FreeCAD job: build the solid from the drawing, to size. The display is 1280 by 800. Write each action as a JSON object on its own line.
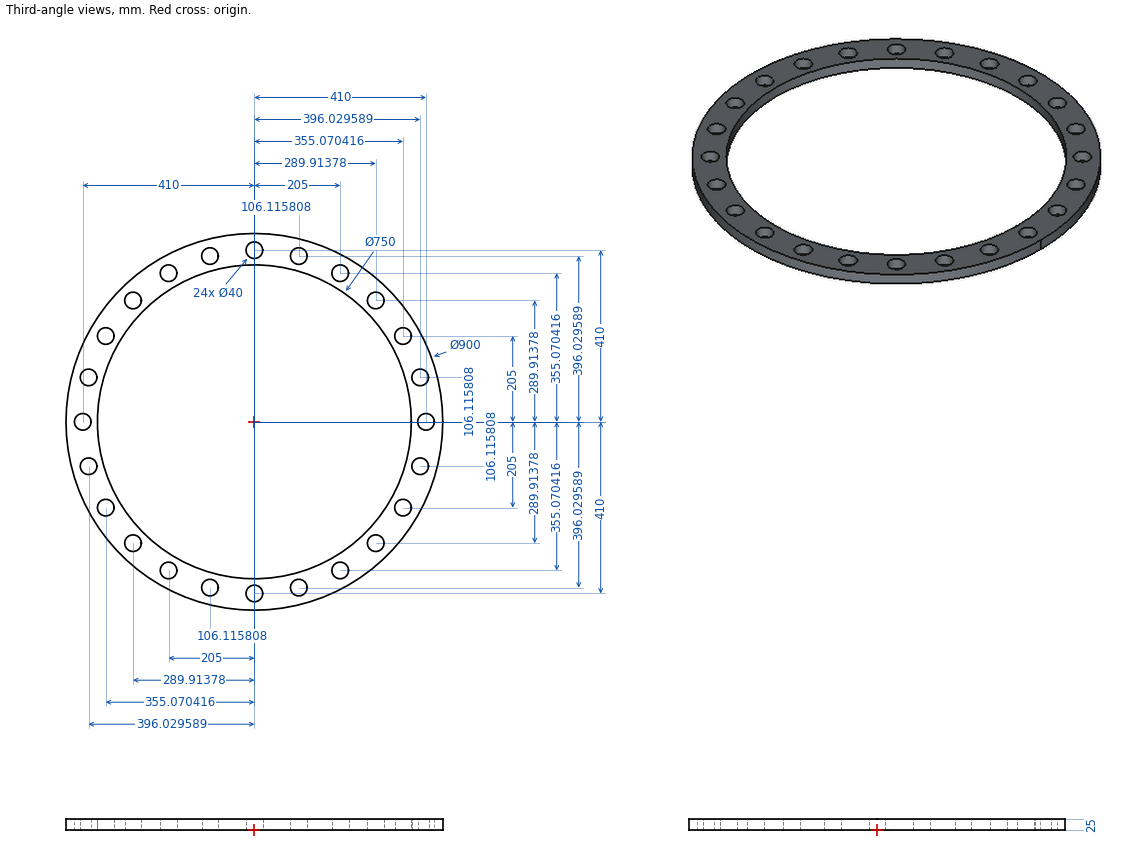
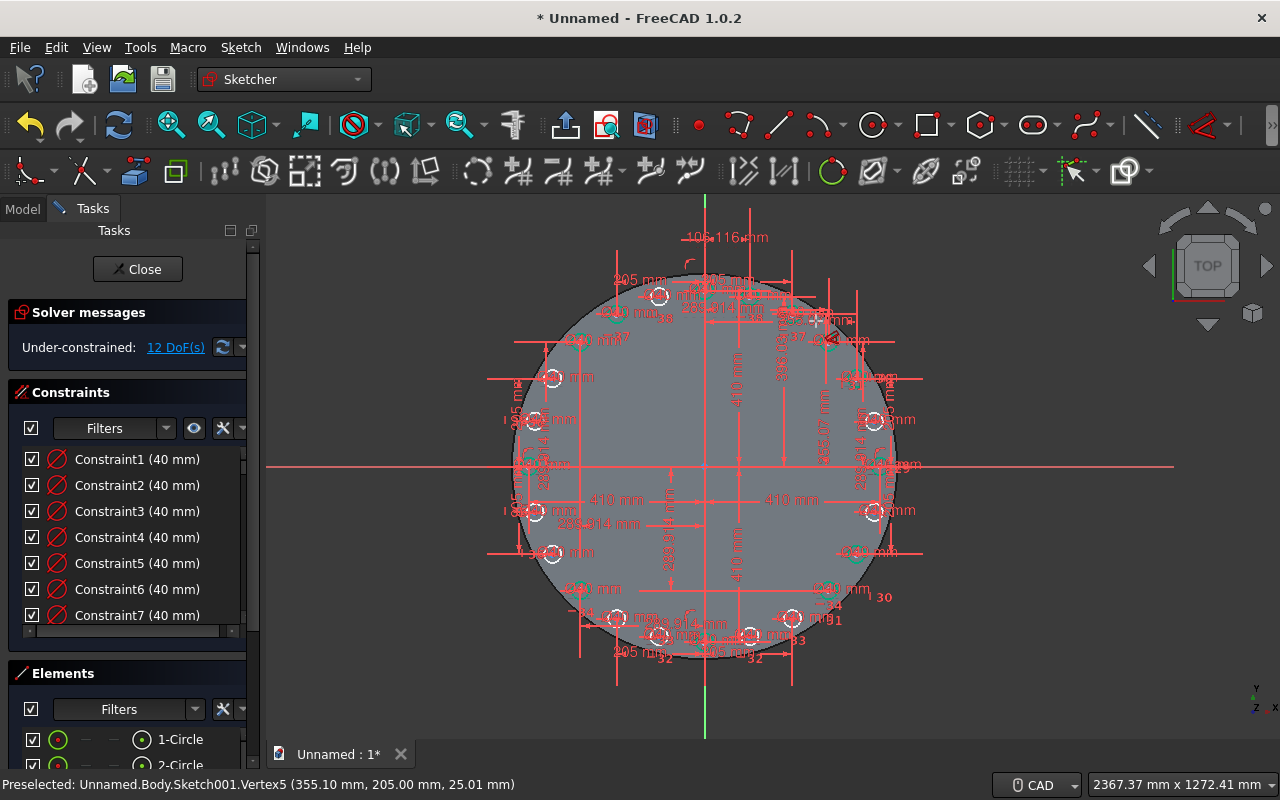
{"action": "left_click", "coordinate": [874, 422]}
{"action": "left_click", "coordinate": [789, 525]}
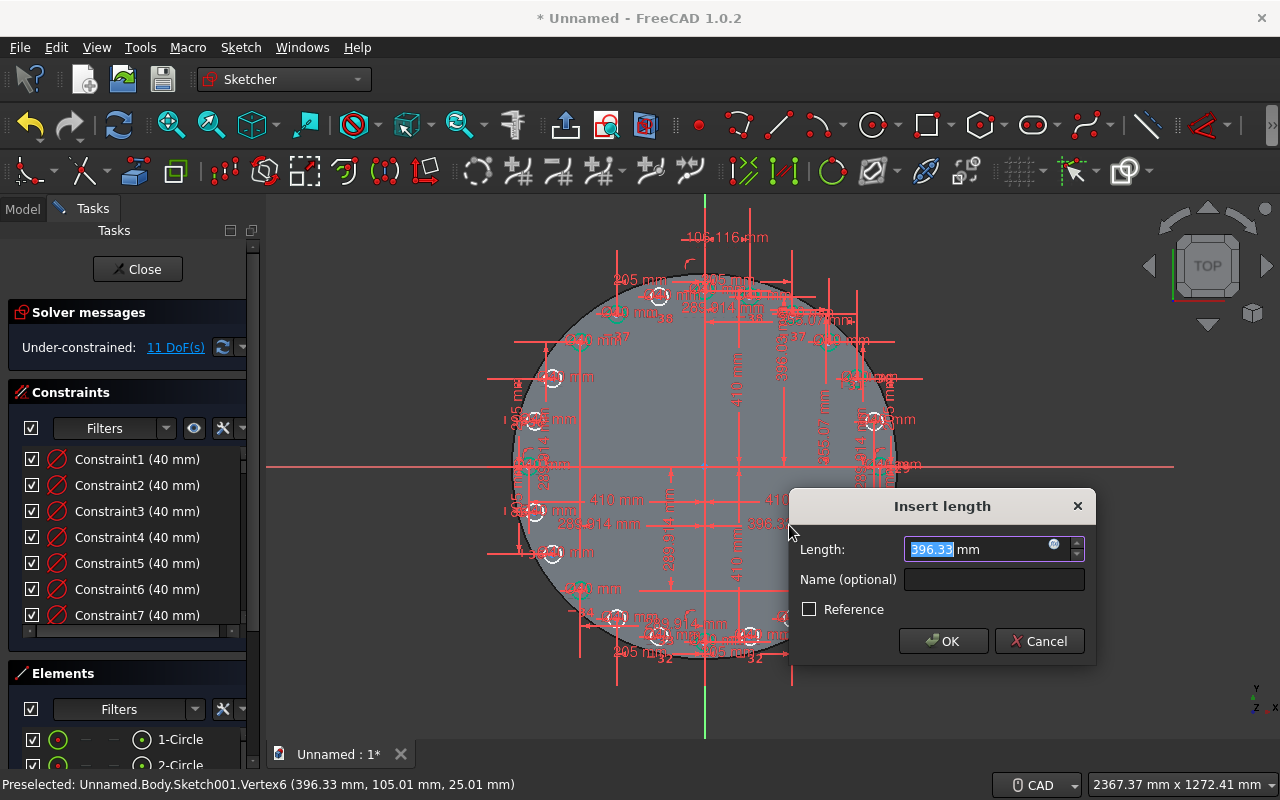
{"action": "type", "text": "396.029589"}
{"action": "key", "text": "Return"}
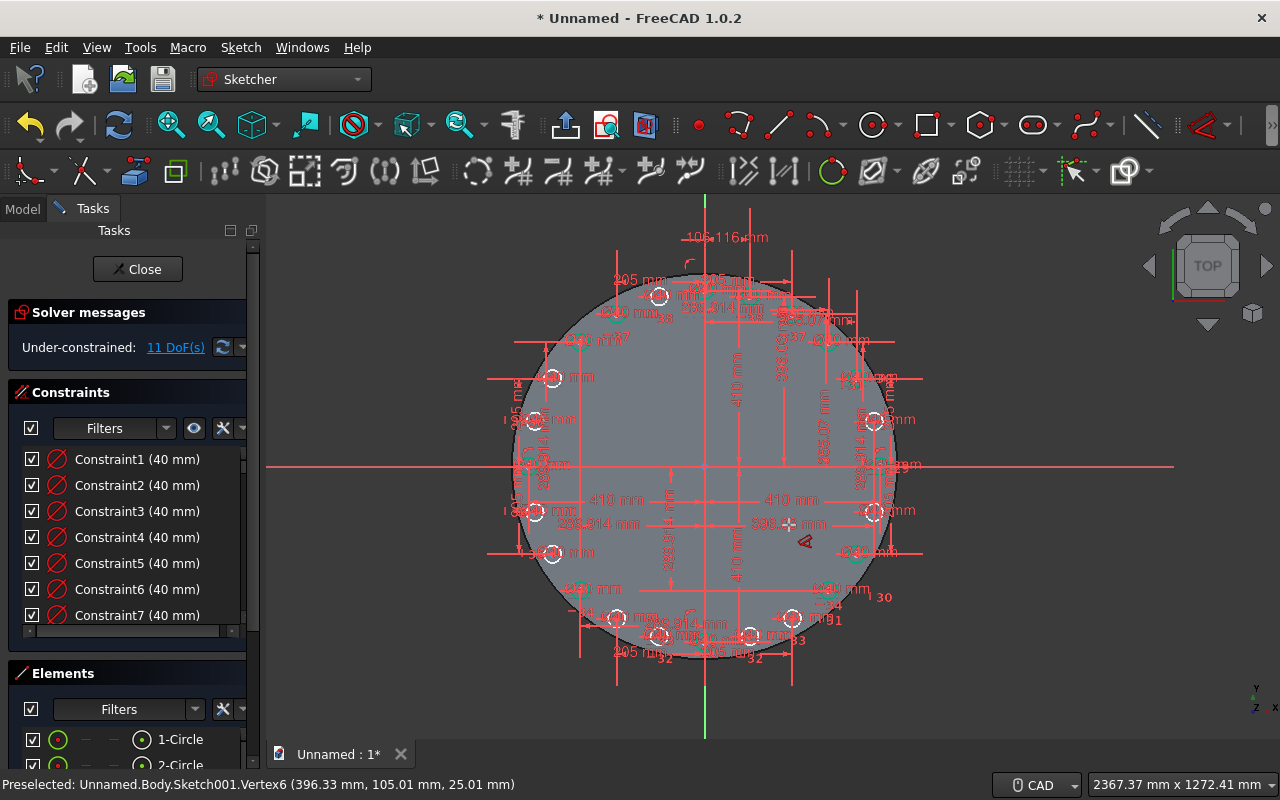
{"action": "left_click", "coordinate": [874, 422]}
{"action": "left_click", "coordinate": [671, 444]}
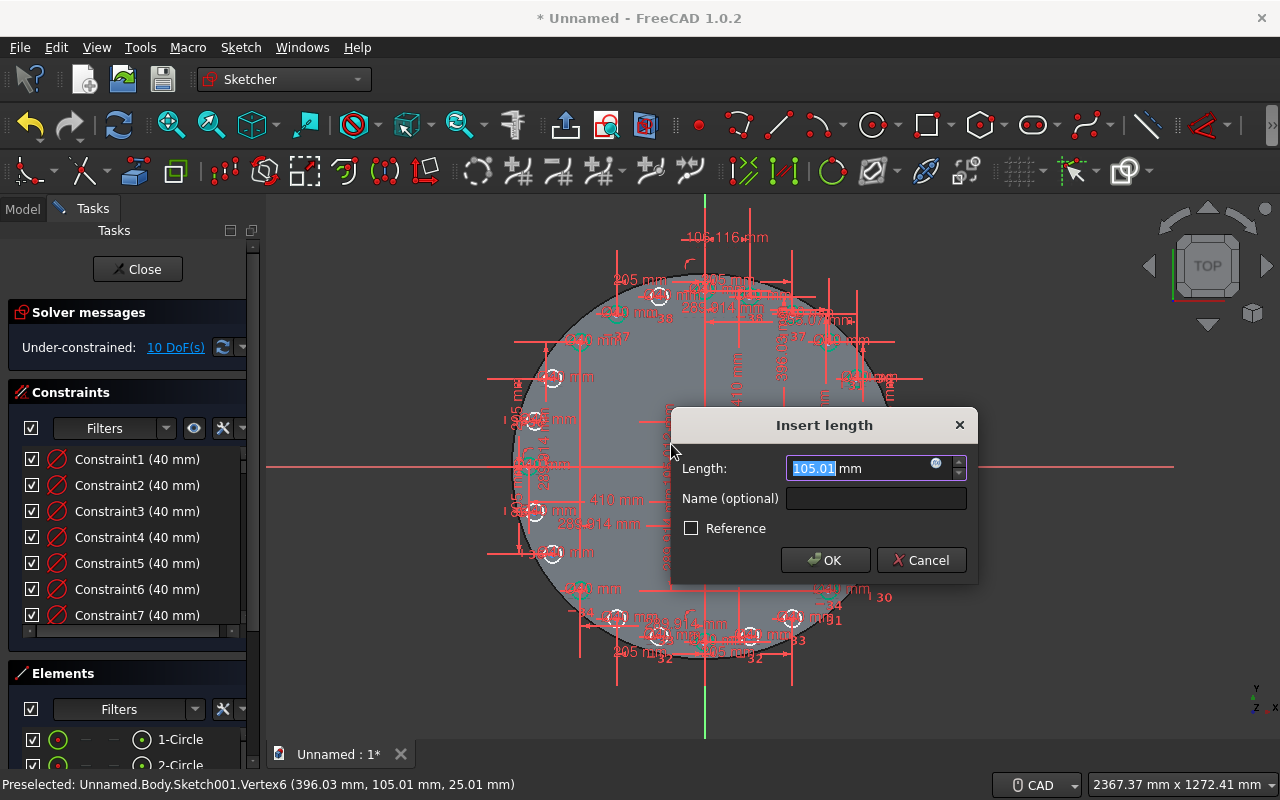
{"action": "type", "text": "106.115808"}
{"action": "key", "text": "Return"}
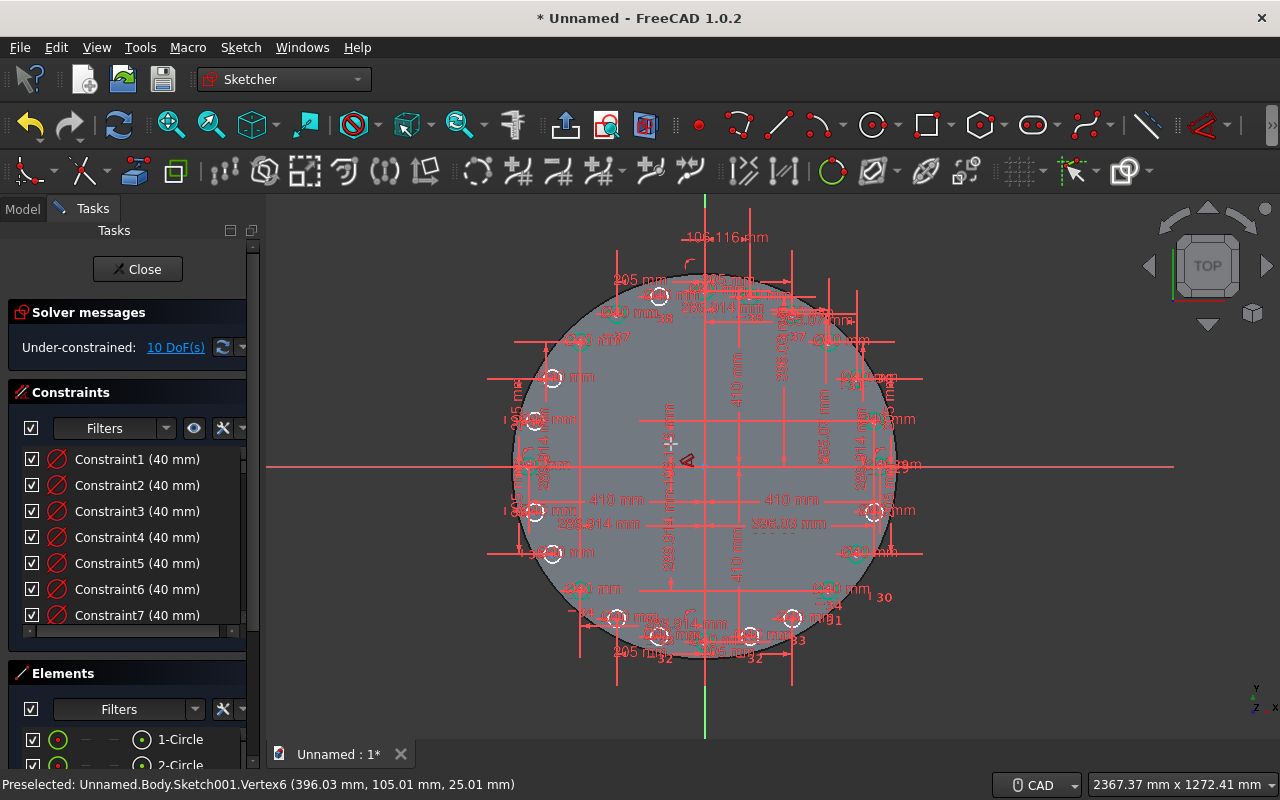
{"action": "left_click", "coordinate": [874, 512]}
{"action": "left_click", "coordinate": [980, 489]}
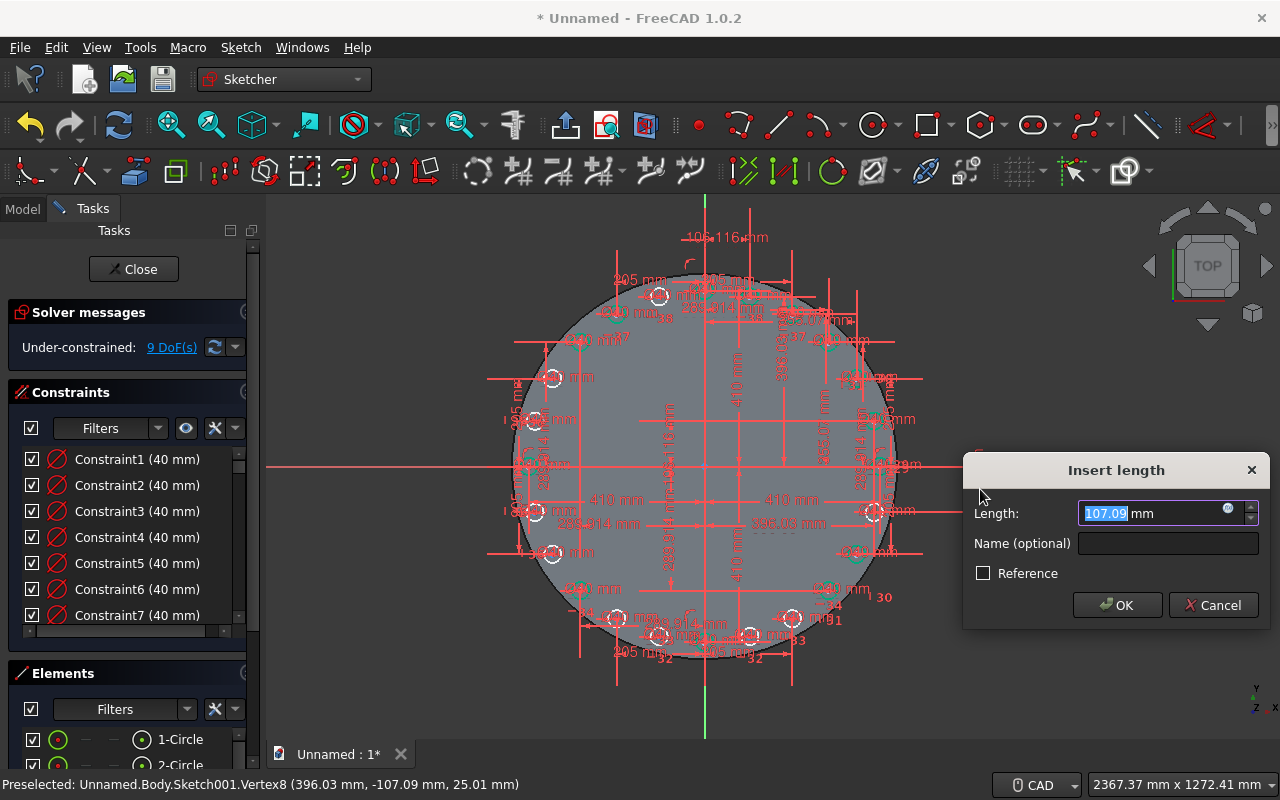
{"action": "type", "text": "106.115808"}
{"action": "key", "text": "Return"}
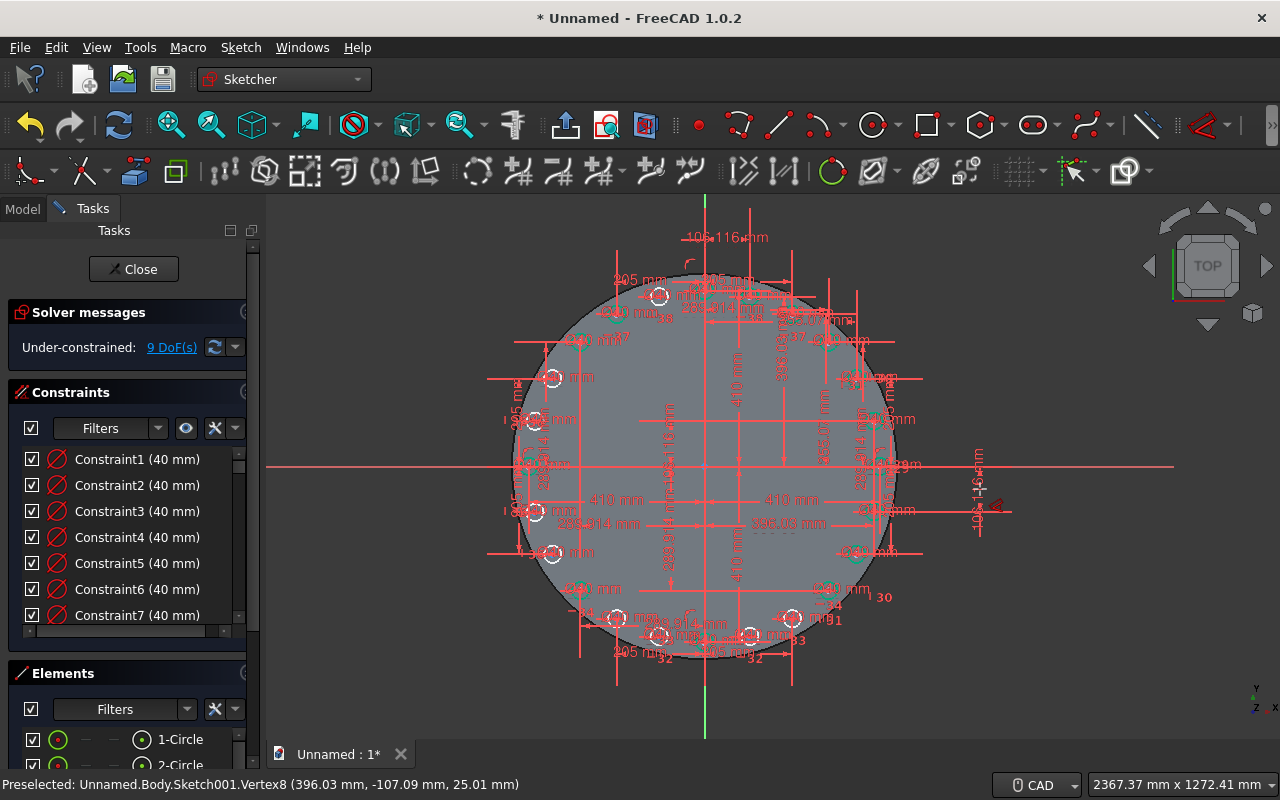
{"action": "left_click", "coordinate": [792, 619]}
{"action": "left_click", "coordinate": [671, 578]}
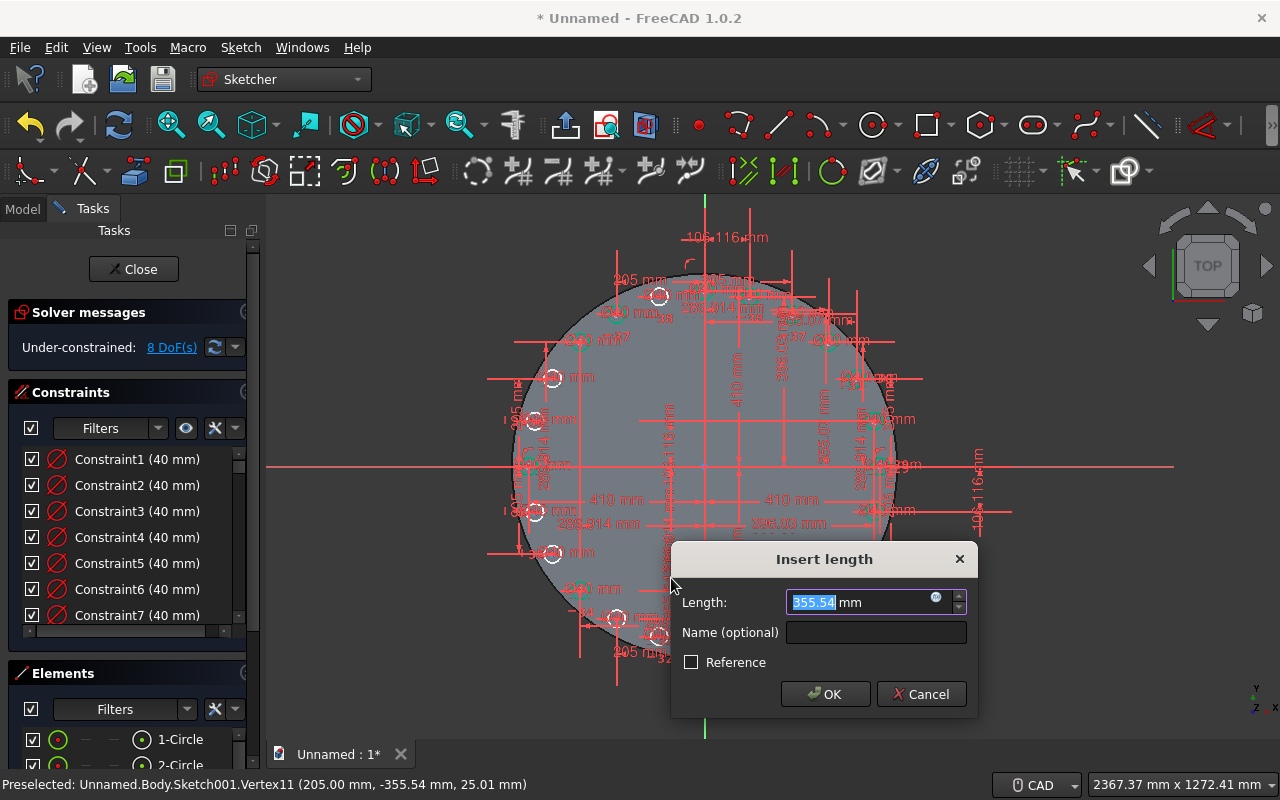
{"action": "type", "text": "355.070416"}
{"action": "key", "text": "Return"}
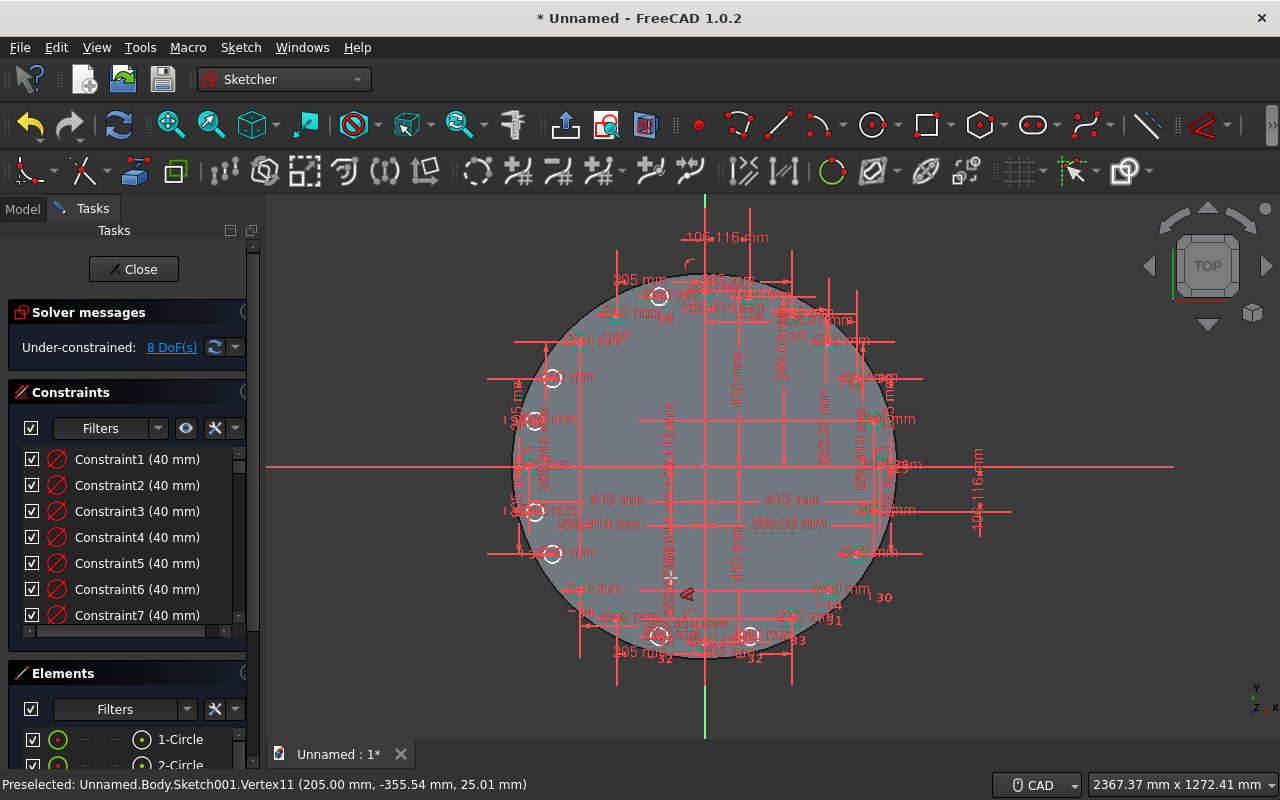
{"action": "left_click", "coordinate": [750, 637]}
{"action": "left_click", "coordinate": [743, 433]}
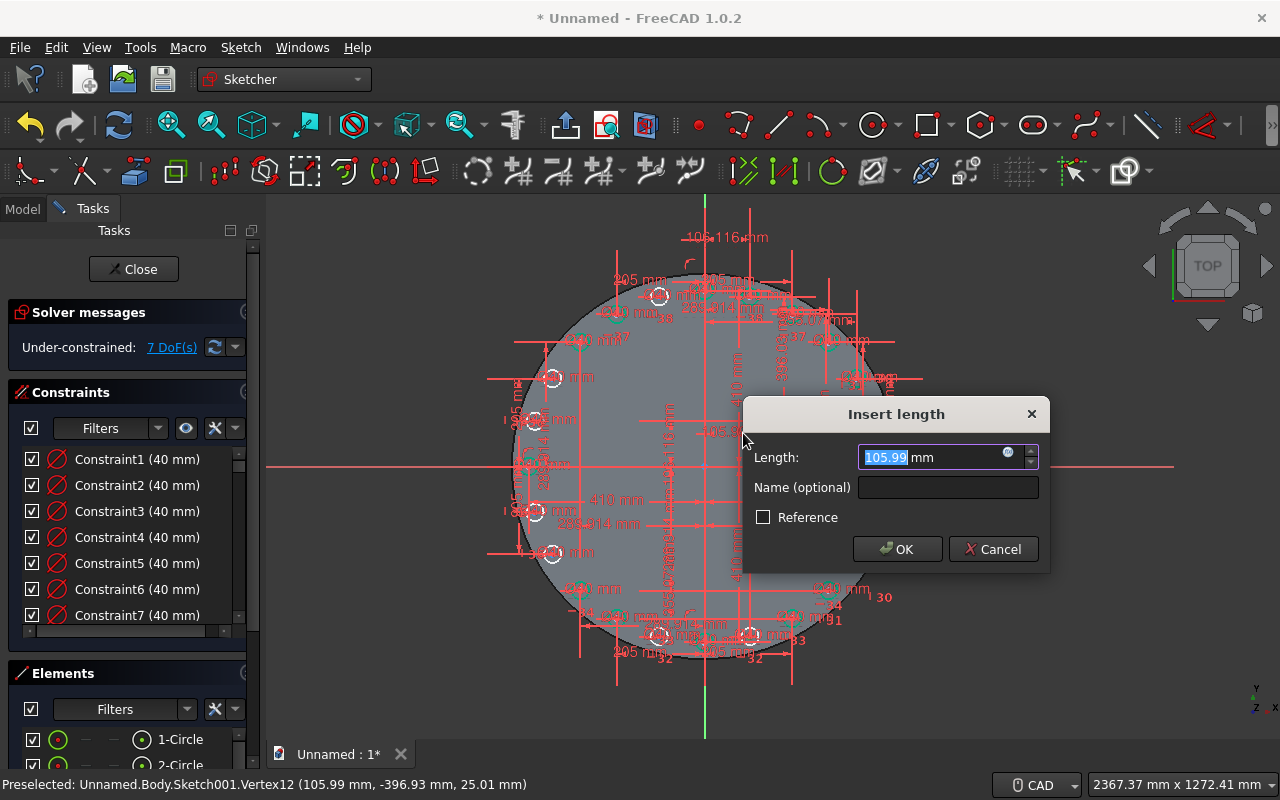
{"action": "type", "text": "106.115808"}
{"action": "key", "text": "Return"}